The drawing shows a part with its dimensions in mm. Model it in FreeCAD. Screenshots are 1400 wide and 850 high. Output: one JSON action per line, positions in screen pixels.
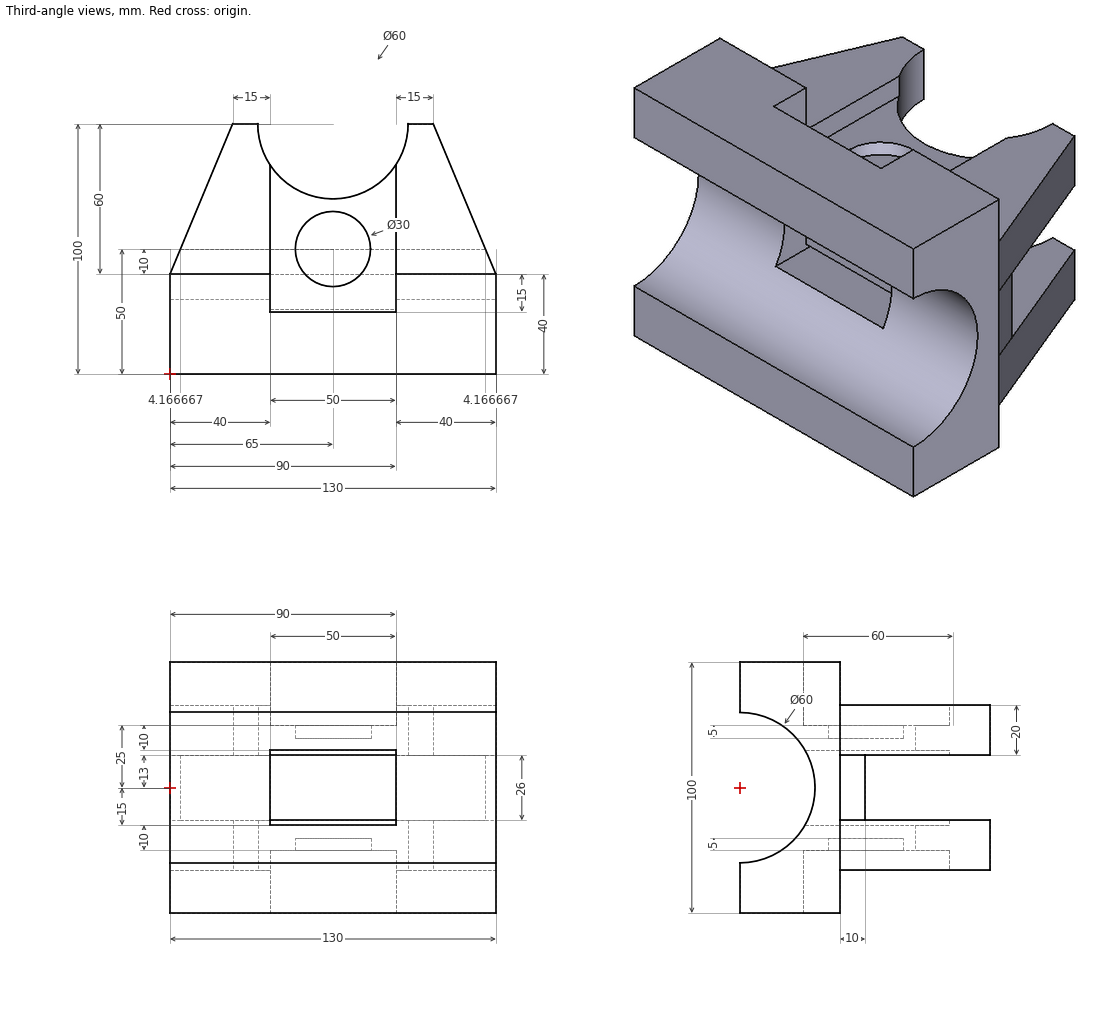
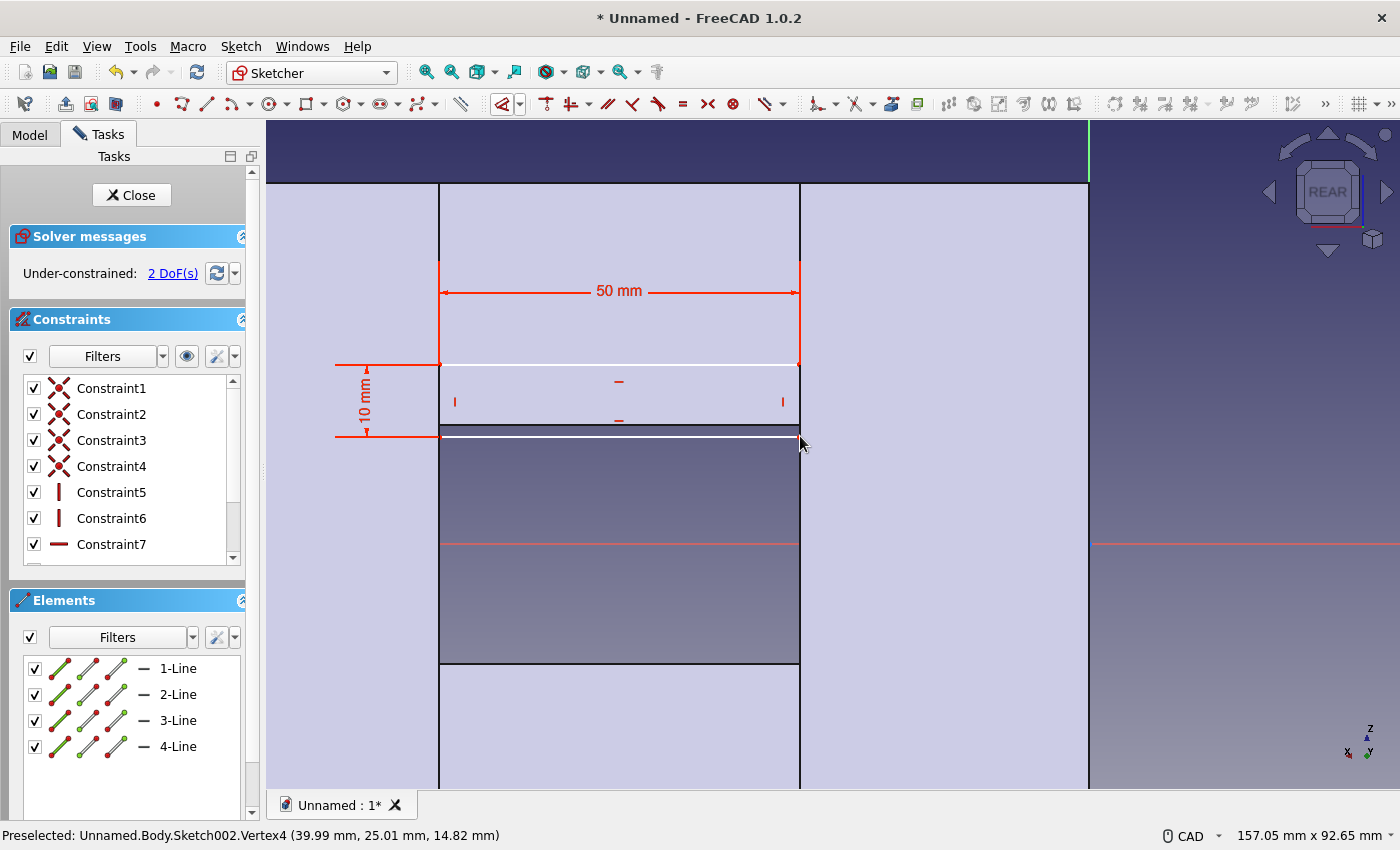
{"action": "left_click", "coordinate": [439, 365]}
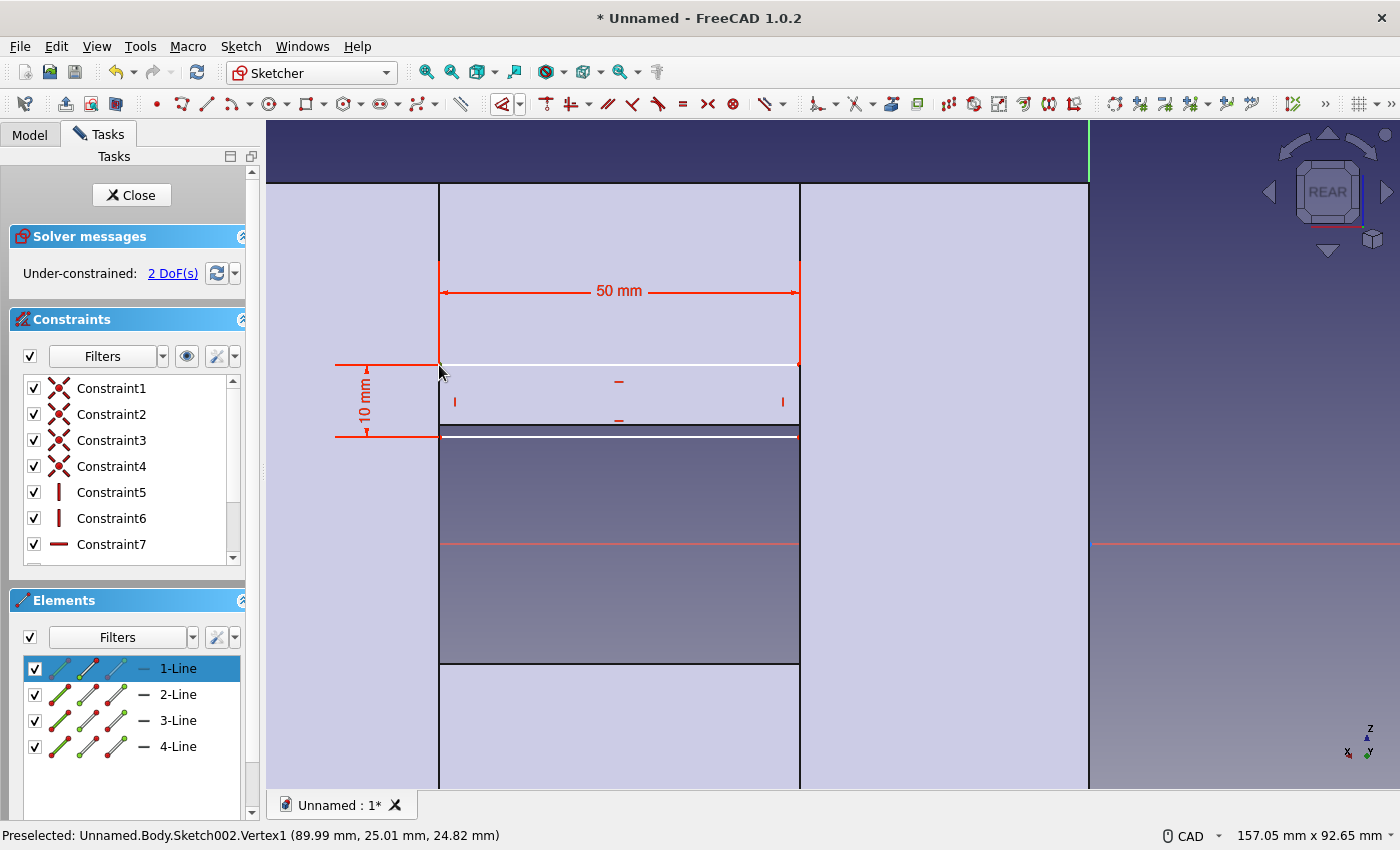
{"action": "key", "text": "l"}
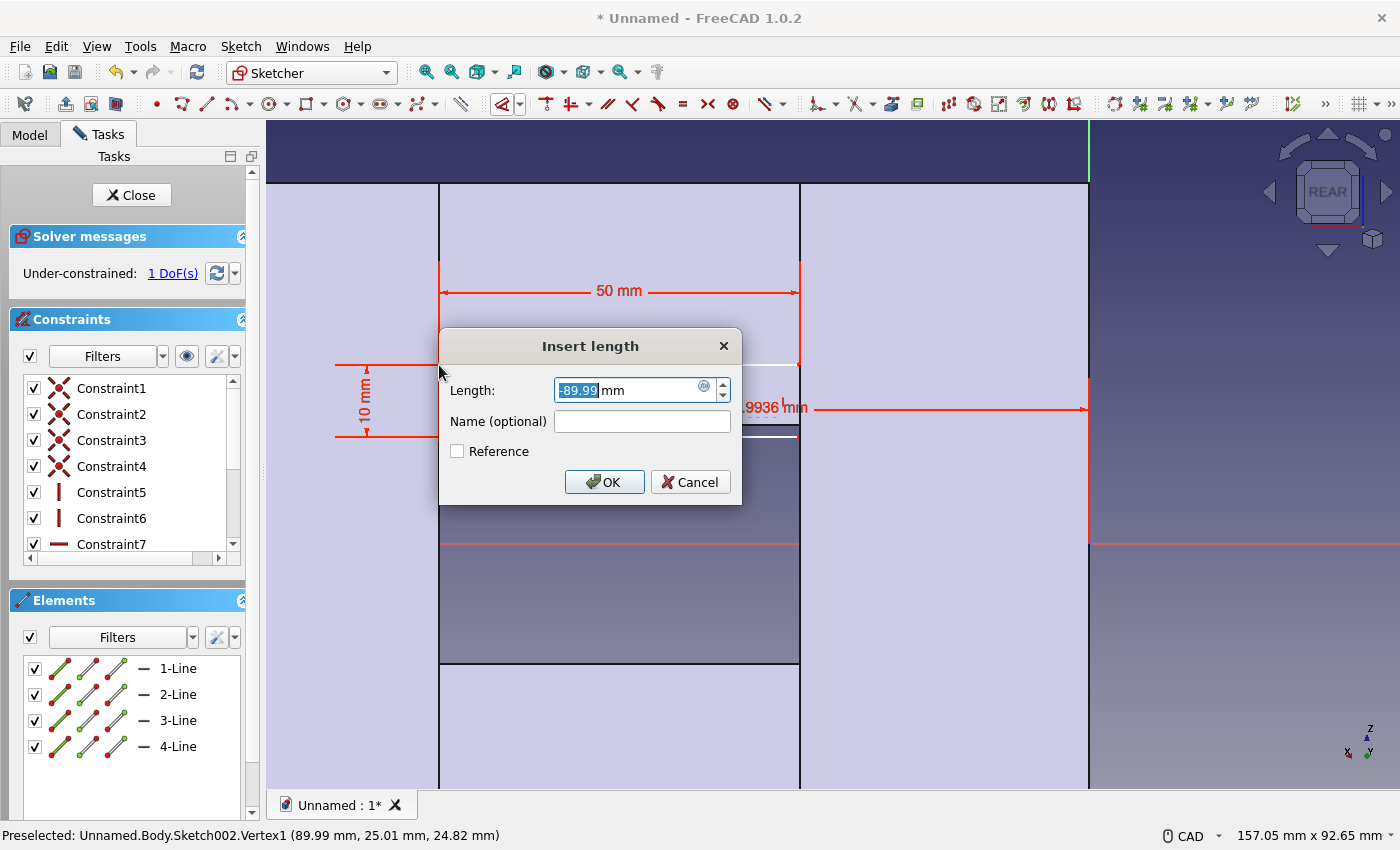
{"action": "type", "text": "-90"}
{"action": "key", "text": "Return"}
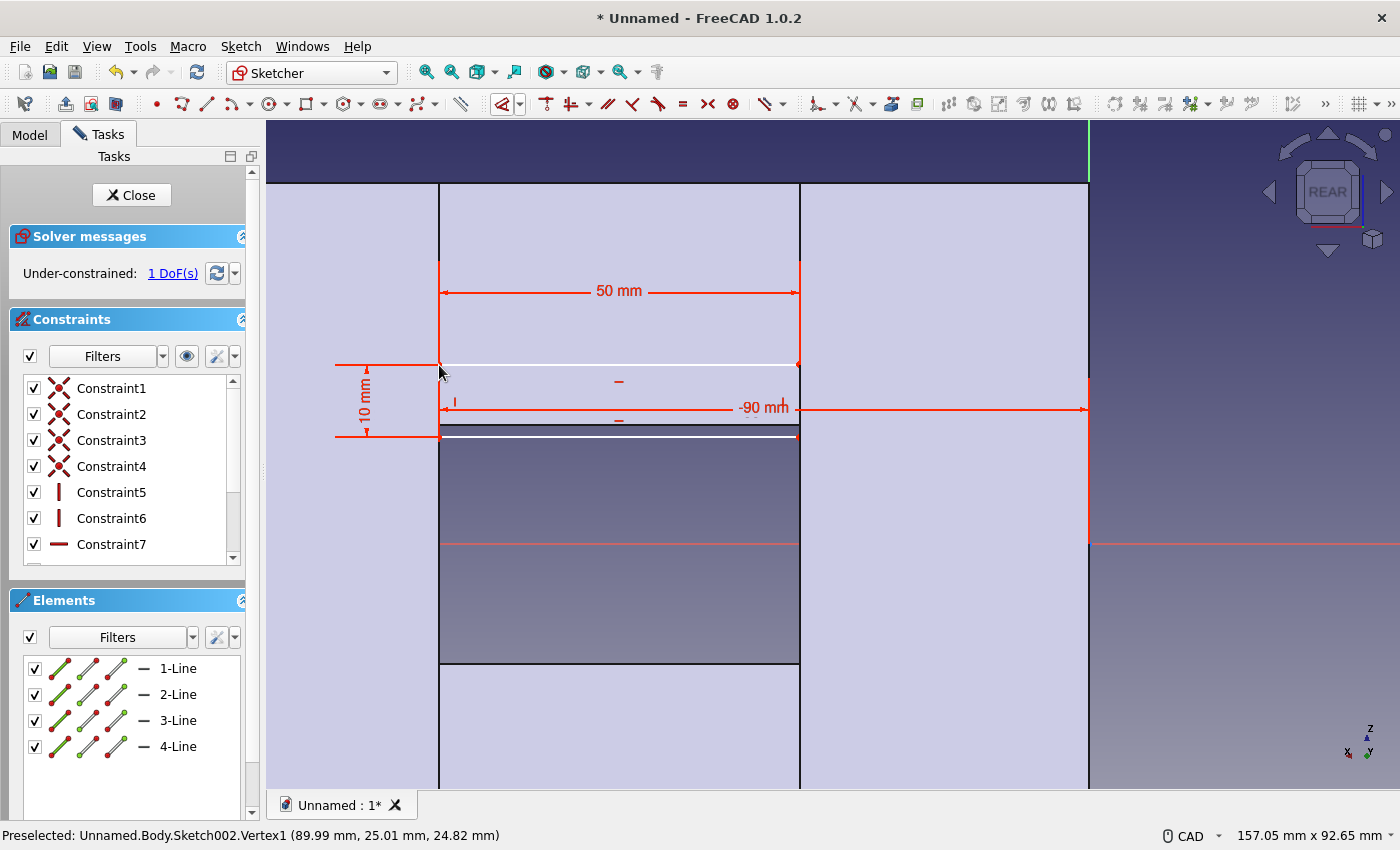
{"action": "left_click", "coordinate": [439, 365]}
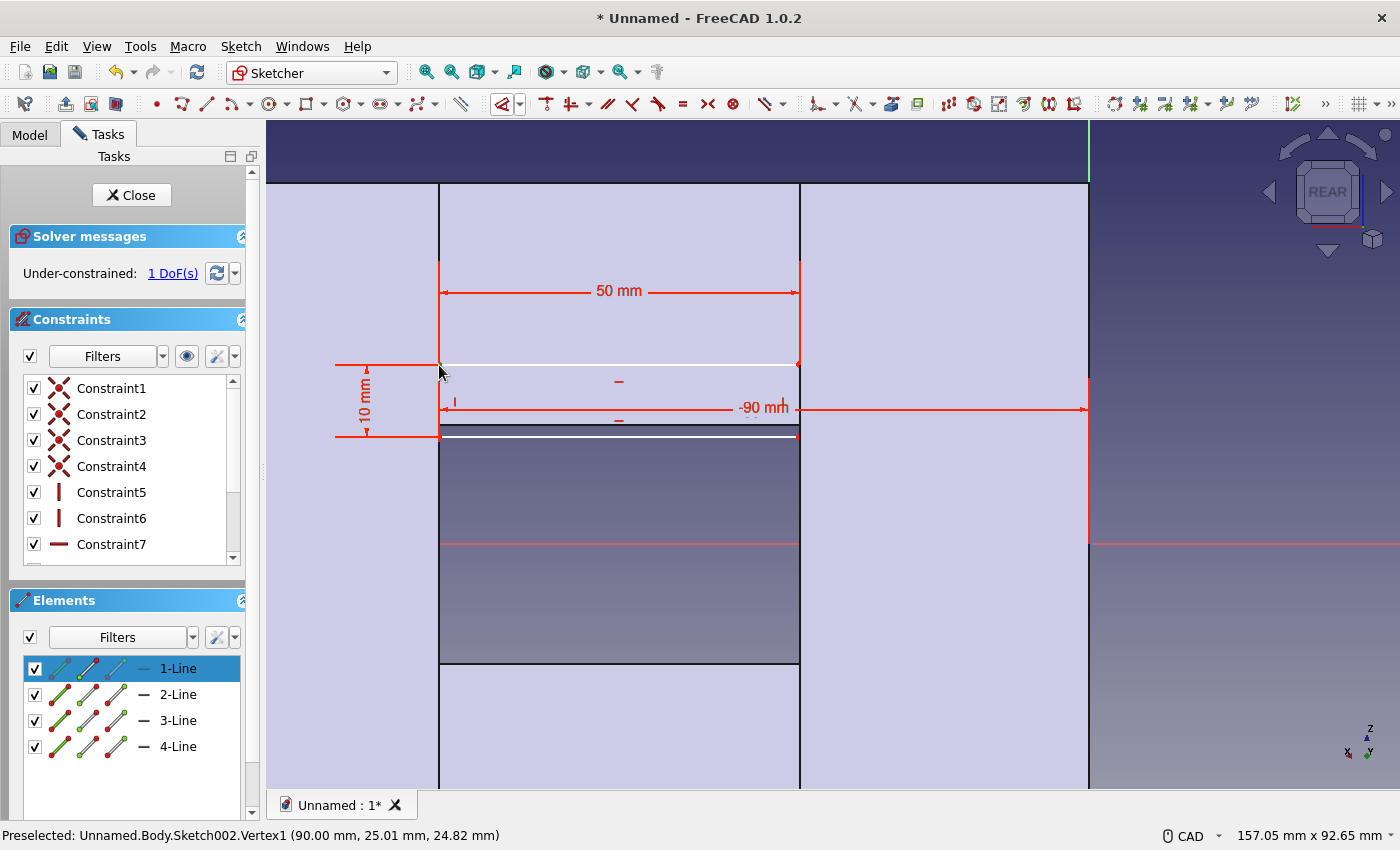
{"action": "left_click", "coordinate": [520, 104]}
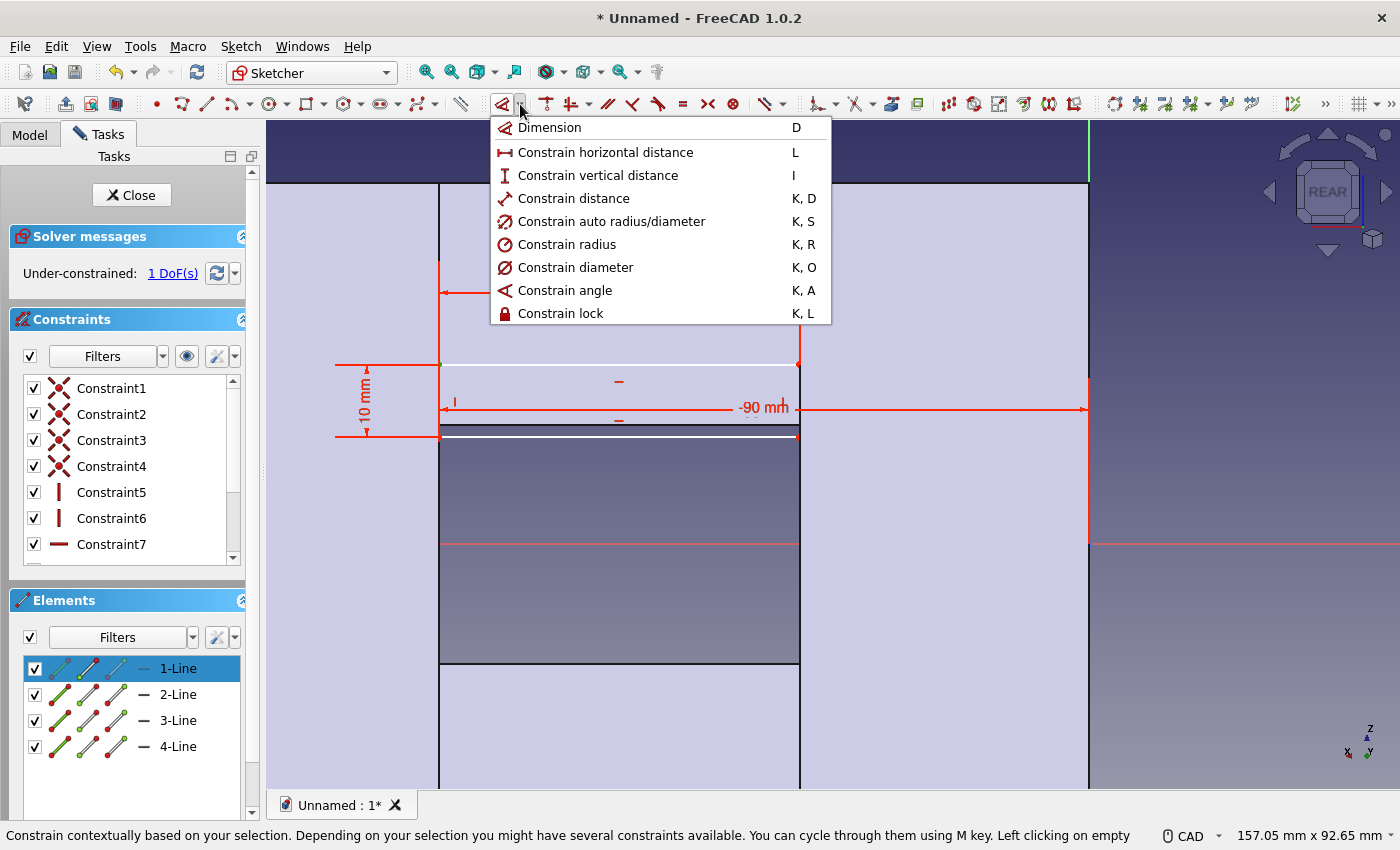
{"action": "left_click", "coordinate": [661, 176]}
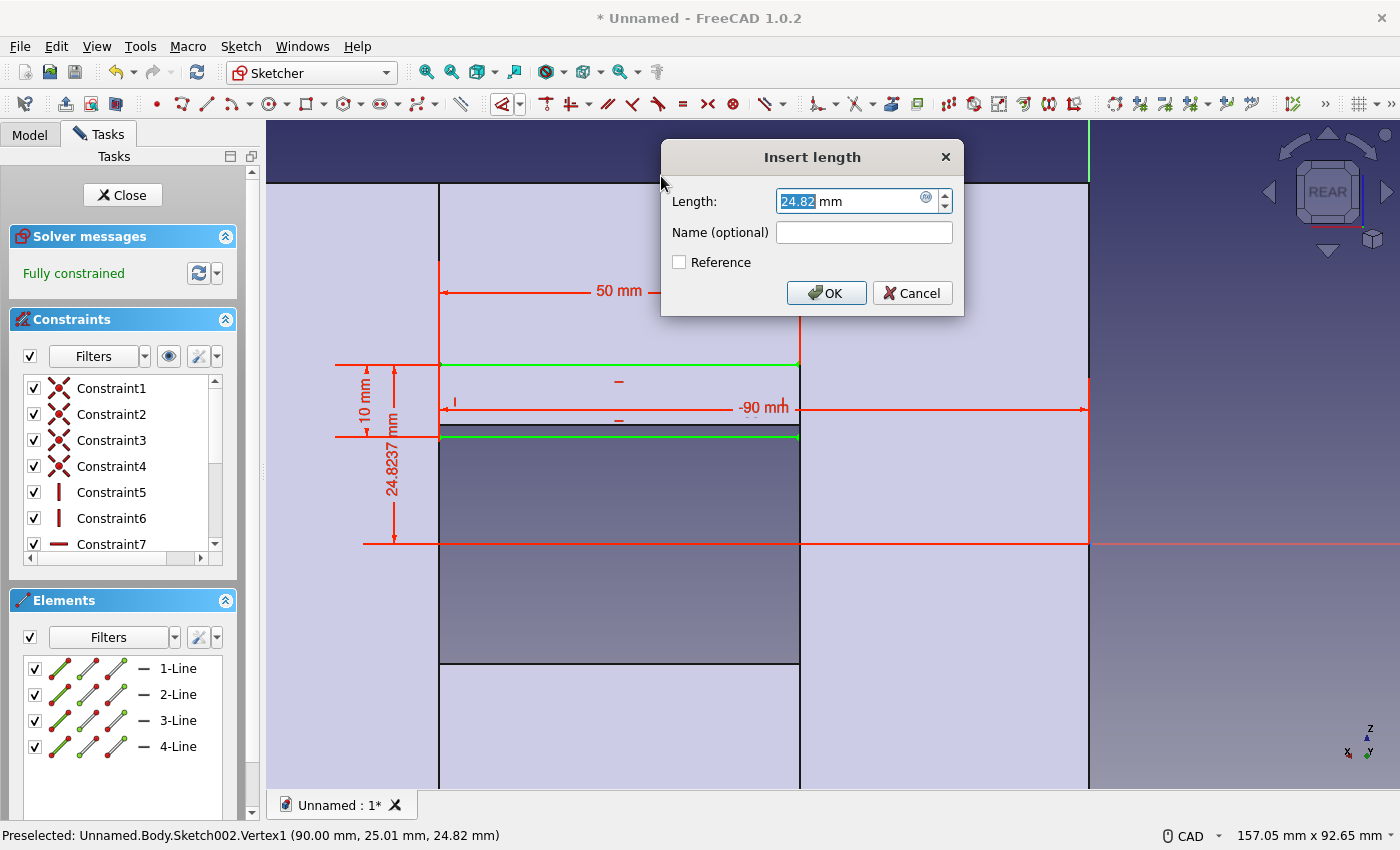
{"action": "type", "text": "25"}
{"action": "key", "text": "Return"}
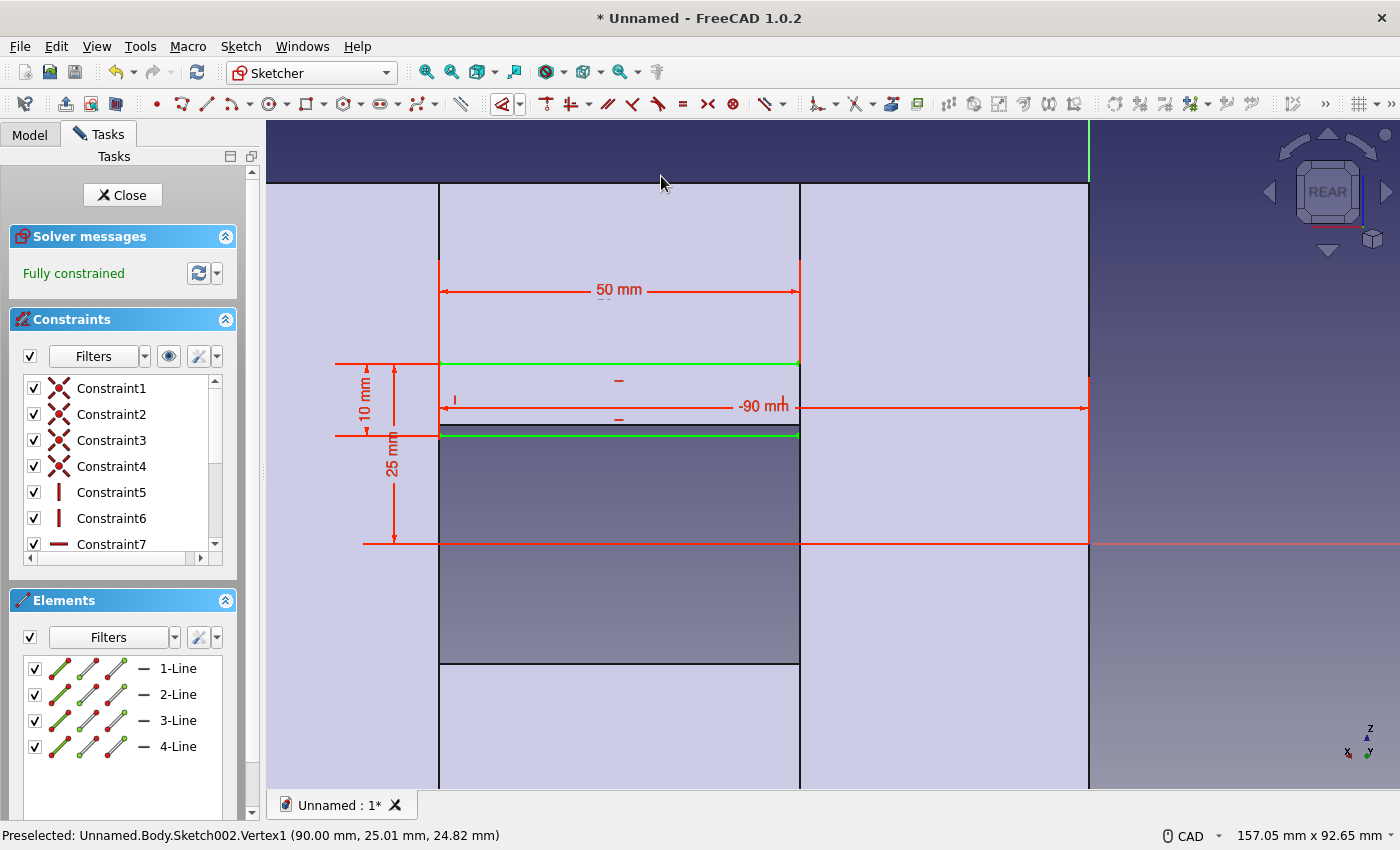
{"action": "left_click", "coordinate": [123, 195]}